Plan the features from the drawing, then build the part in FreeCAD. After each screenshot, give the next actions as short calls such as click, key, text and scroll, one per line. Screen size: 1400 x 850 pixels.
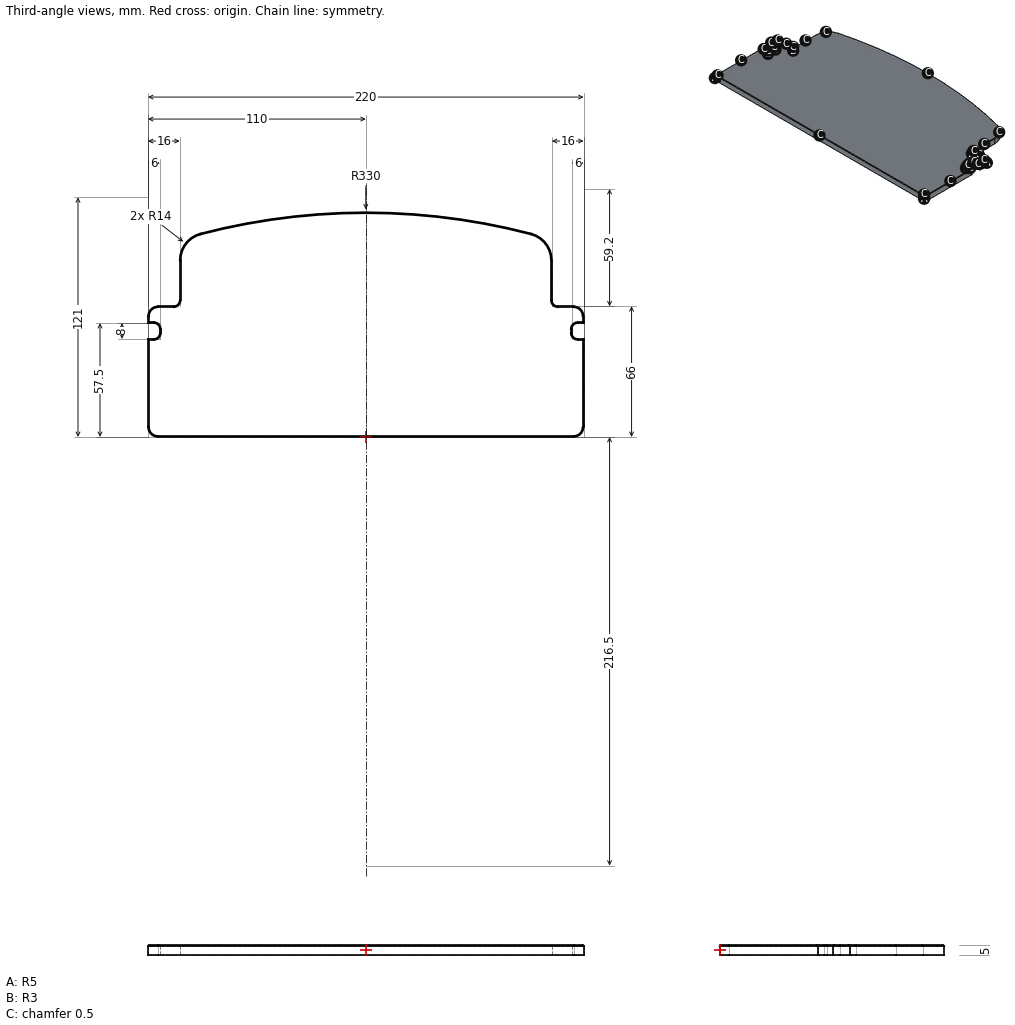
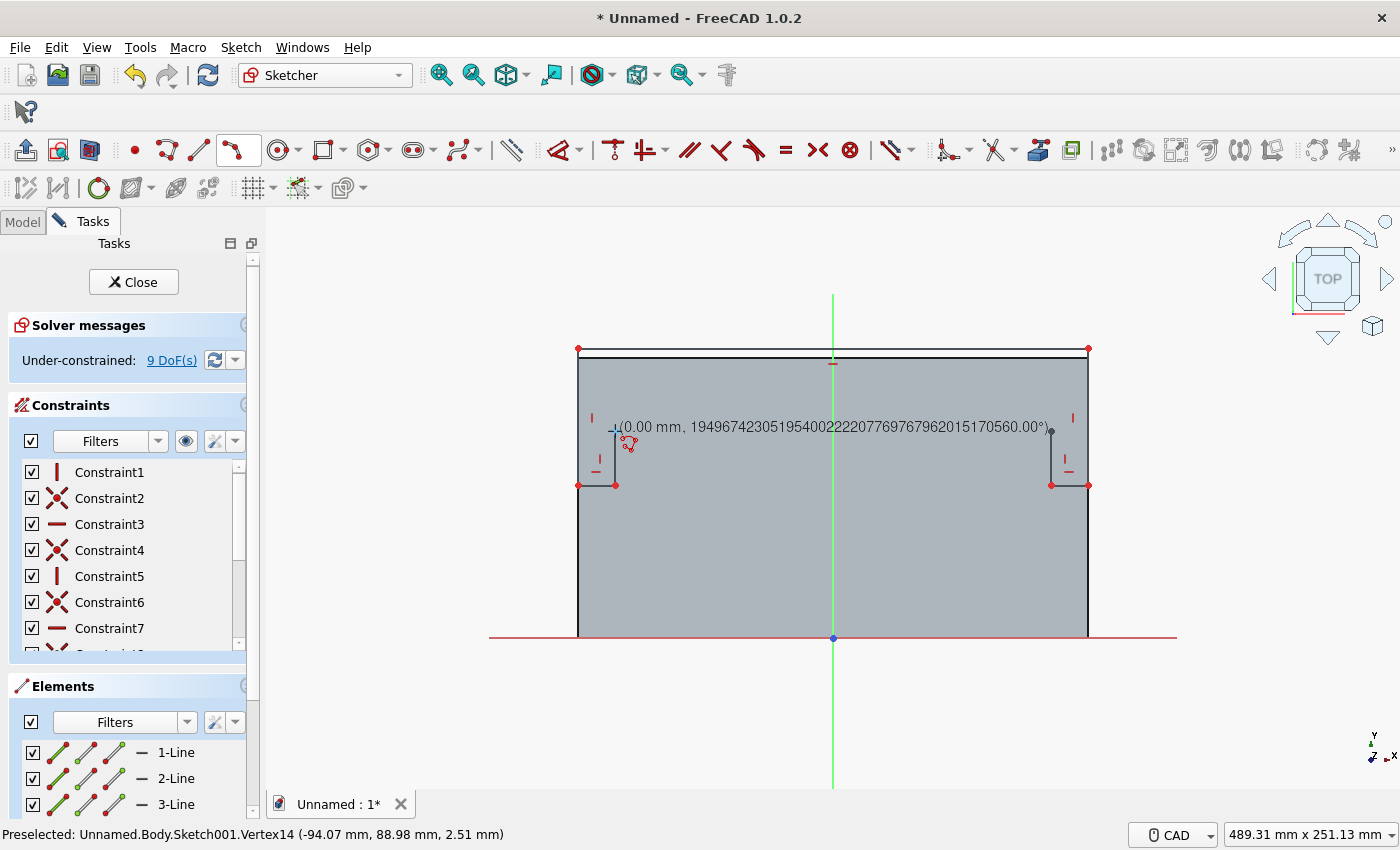
key(g)
key(3)
key(a)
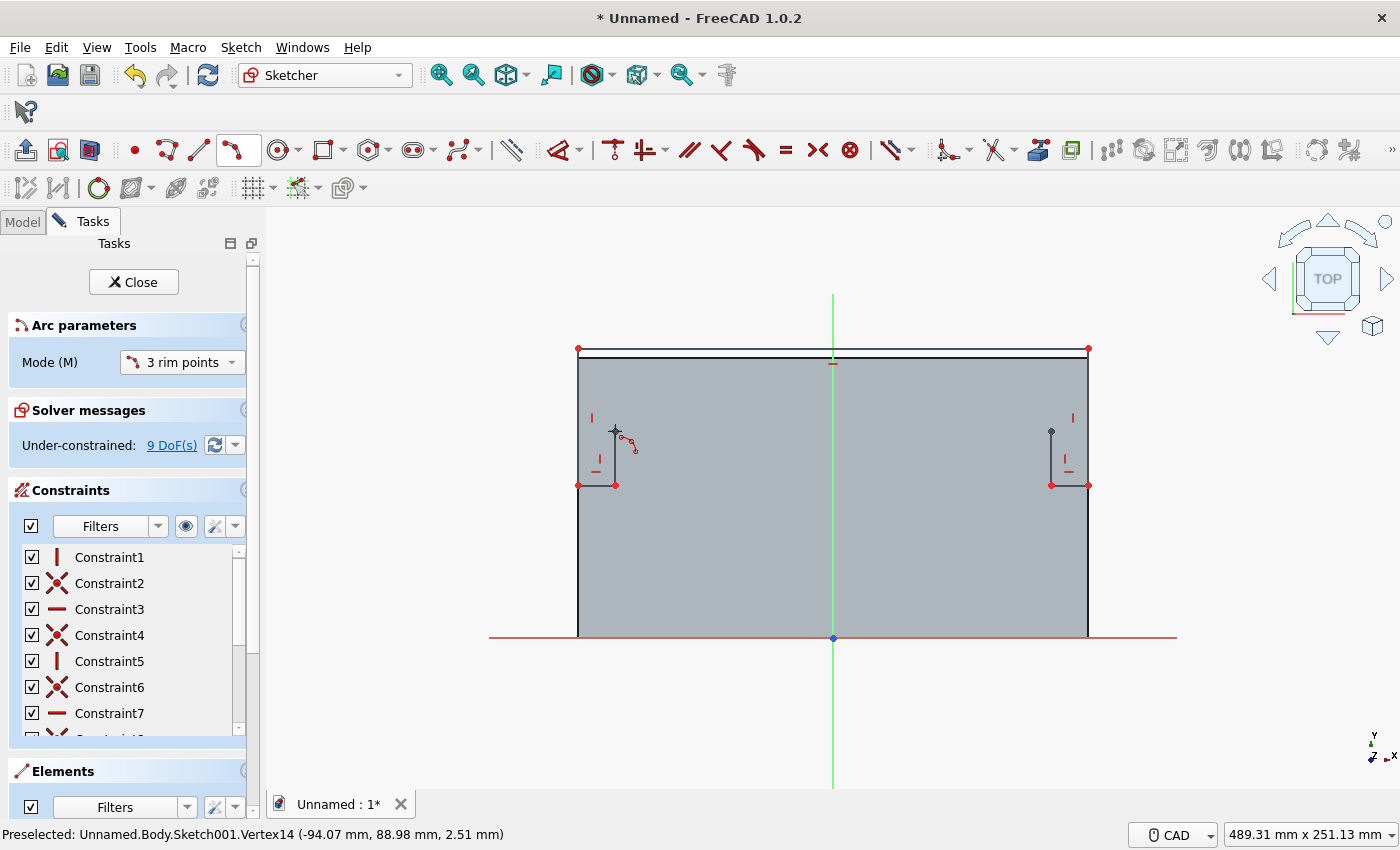
click(615, 432)
click(639, 400)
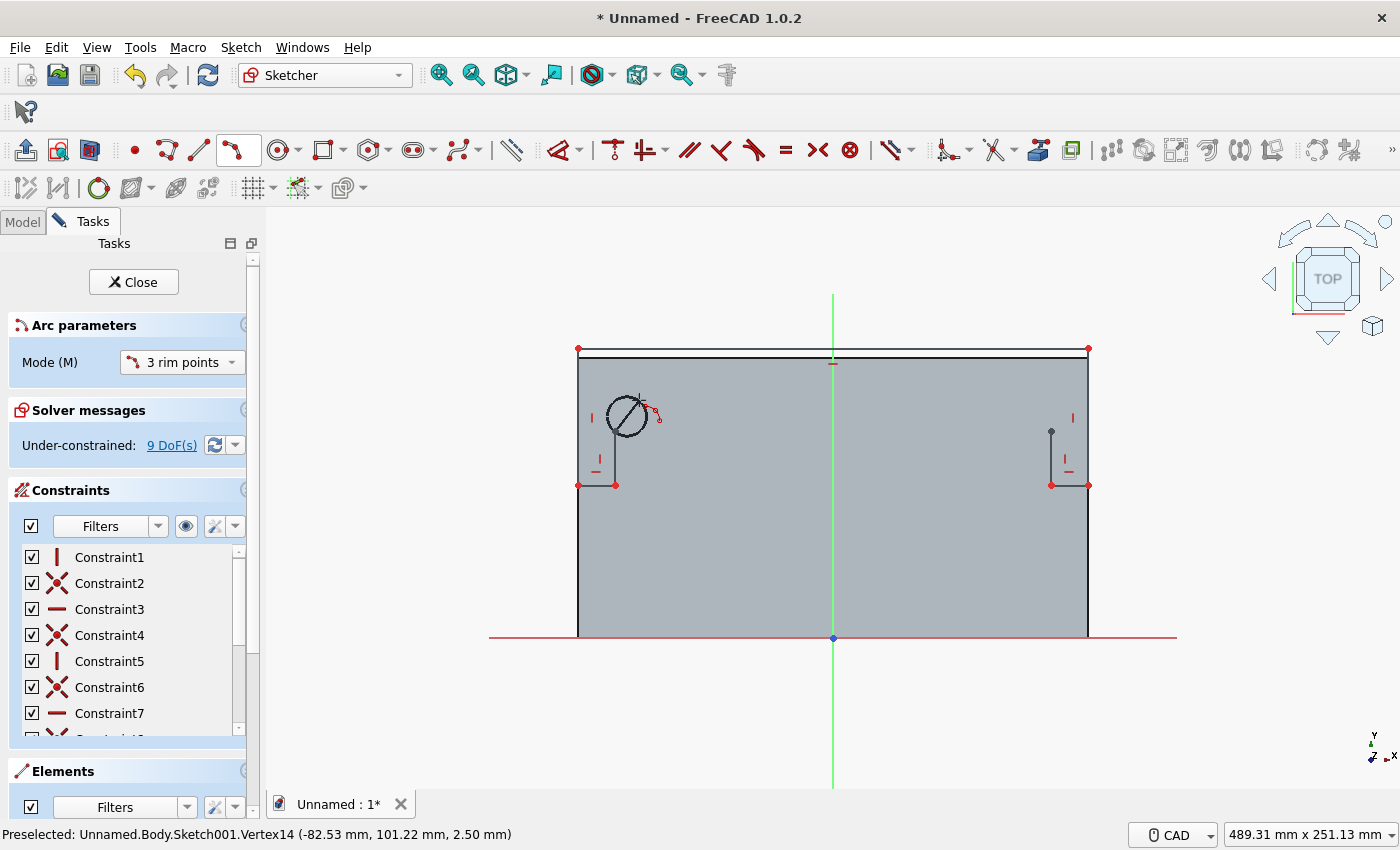
scroll(622, 412, up, 5)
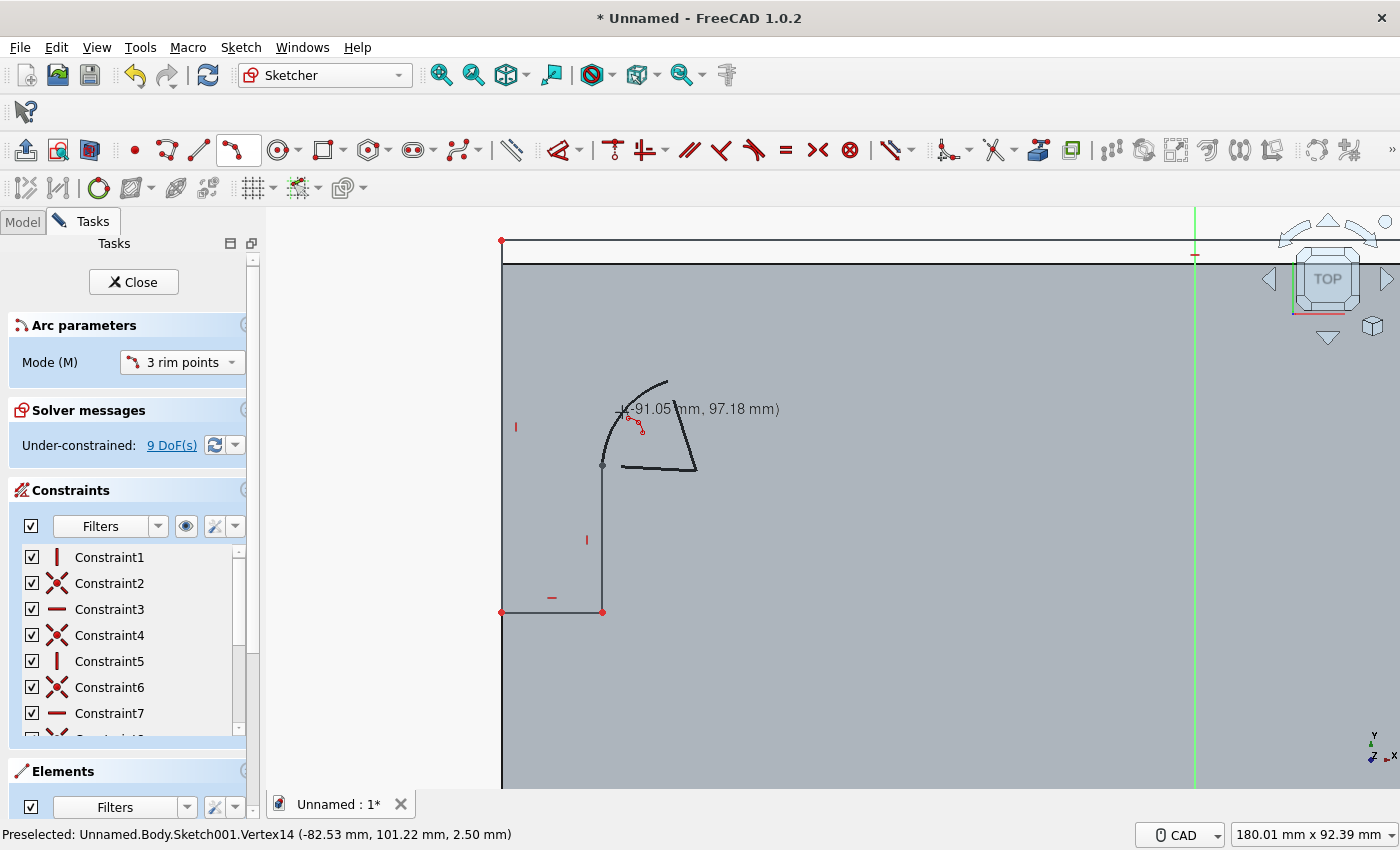
click(621, 410)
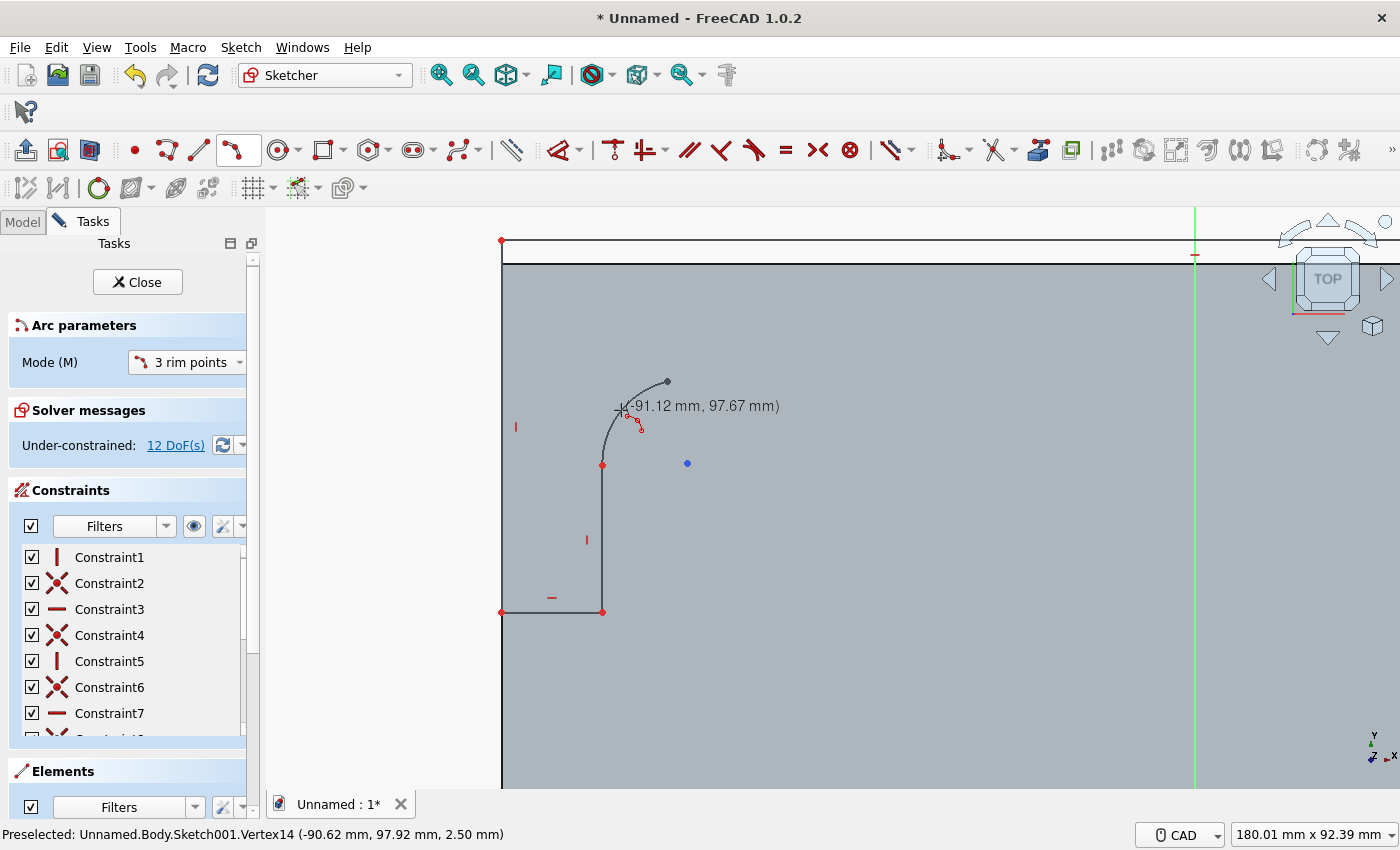
click(668, 381)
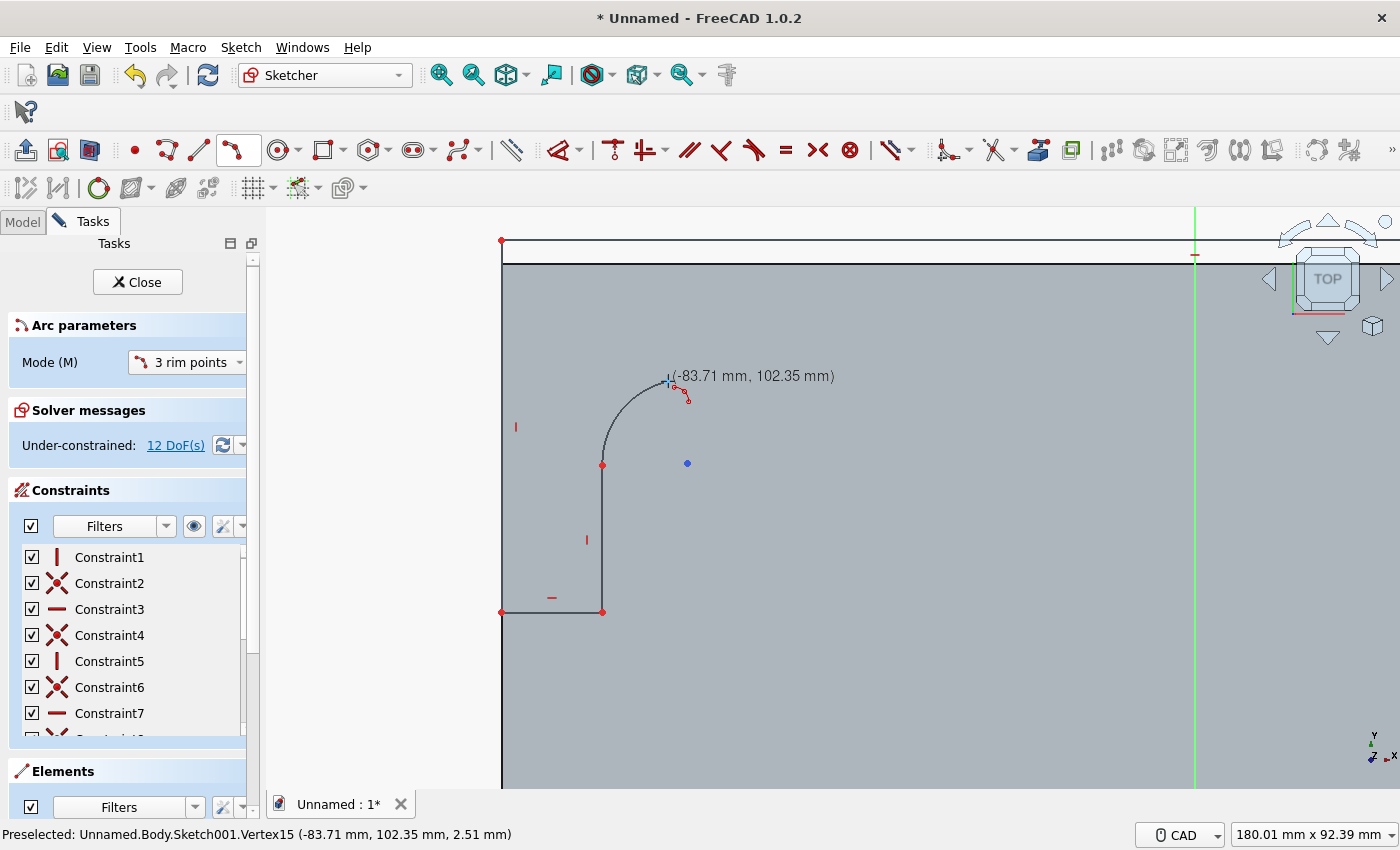
scroll(413, 389, down, 4)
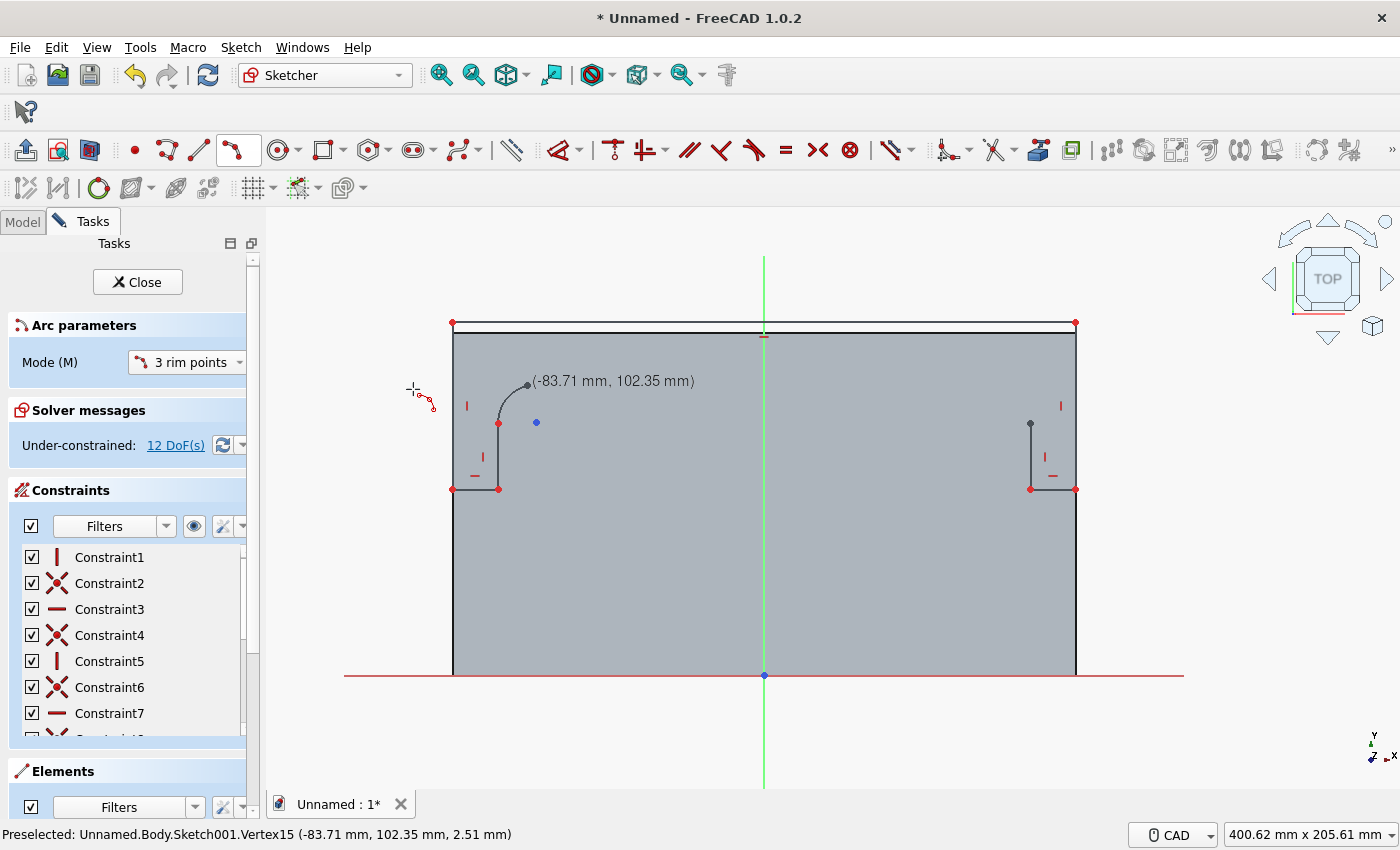
click(1001, 385)
click(812, 355)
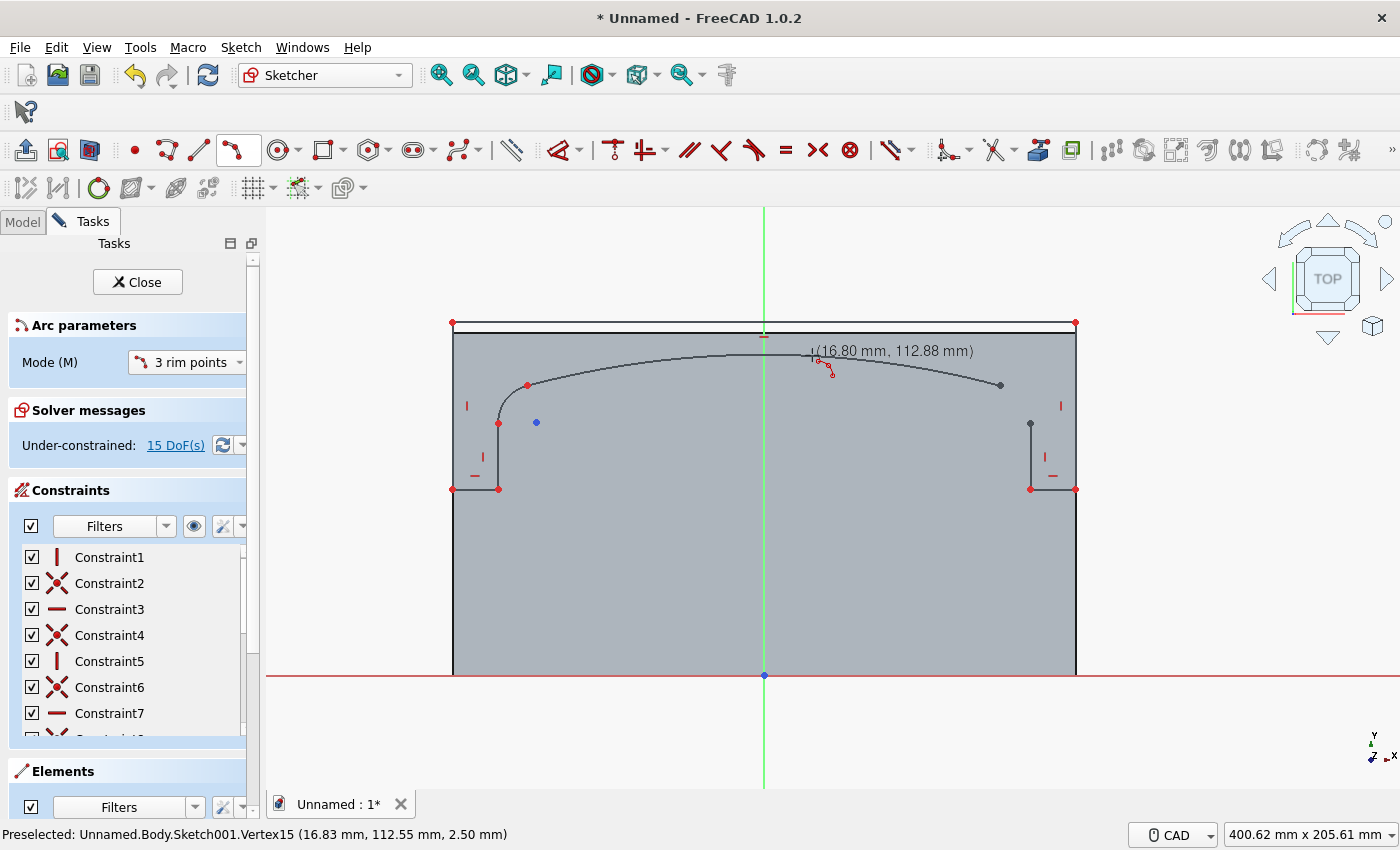
click(1001, 386)
click(1031, 424)